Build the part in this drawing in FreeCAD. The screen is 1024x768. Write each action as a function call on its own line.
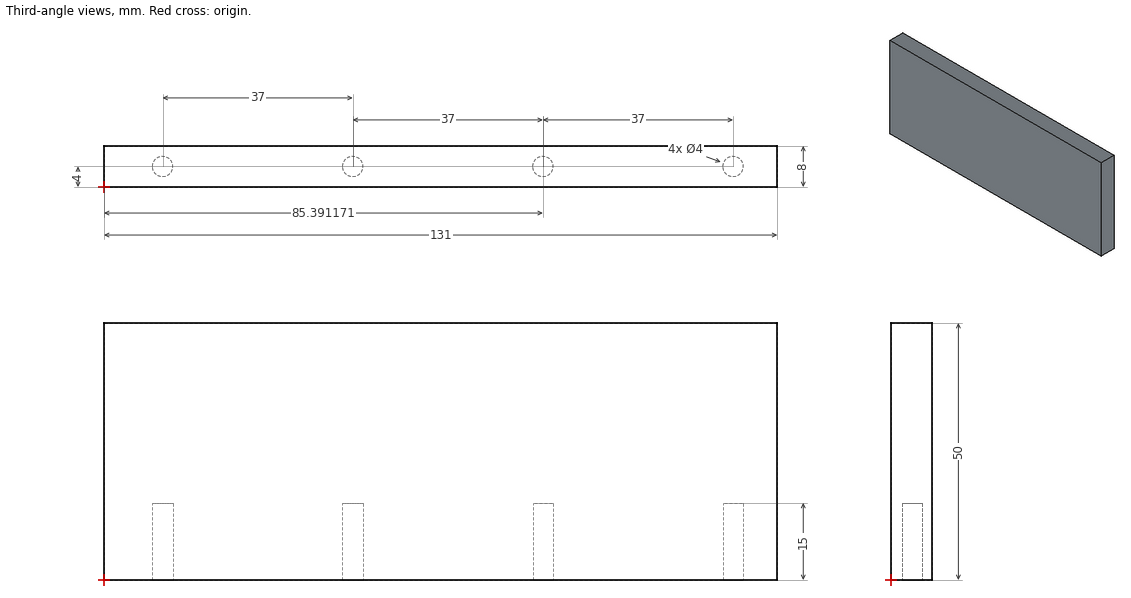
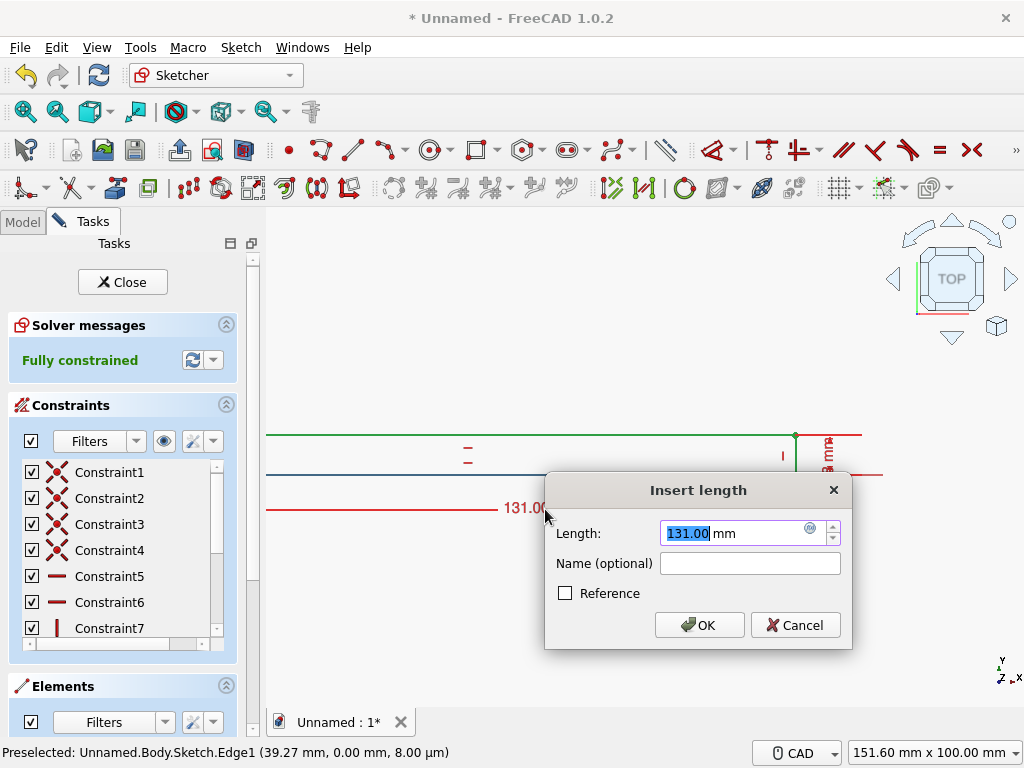
text(131)
key(Return)
key(Escape)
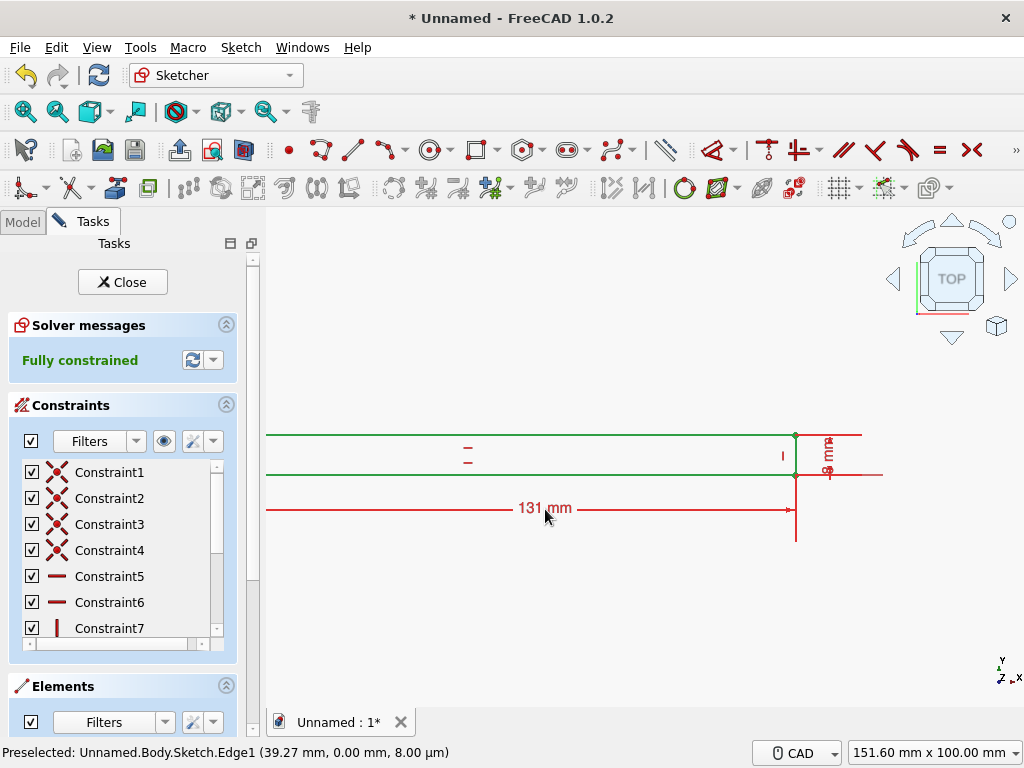
click(123, 282)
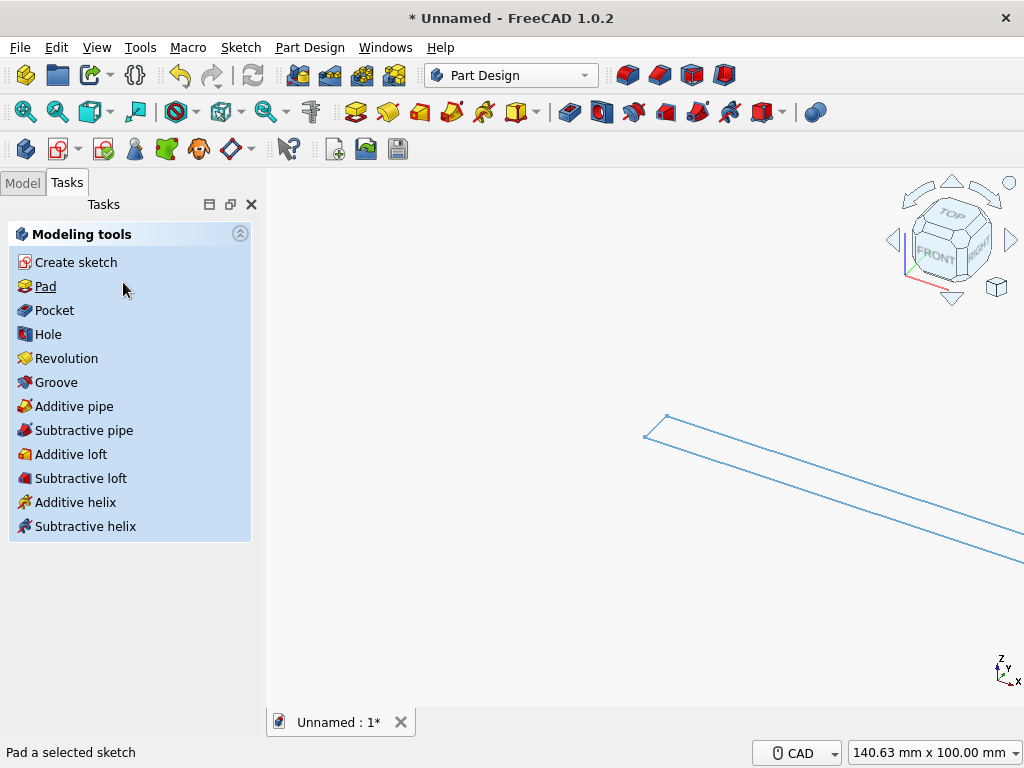
click(356, 112)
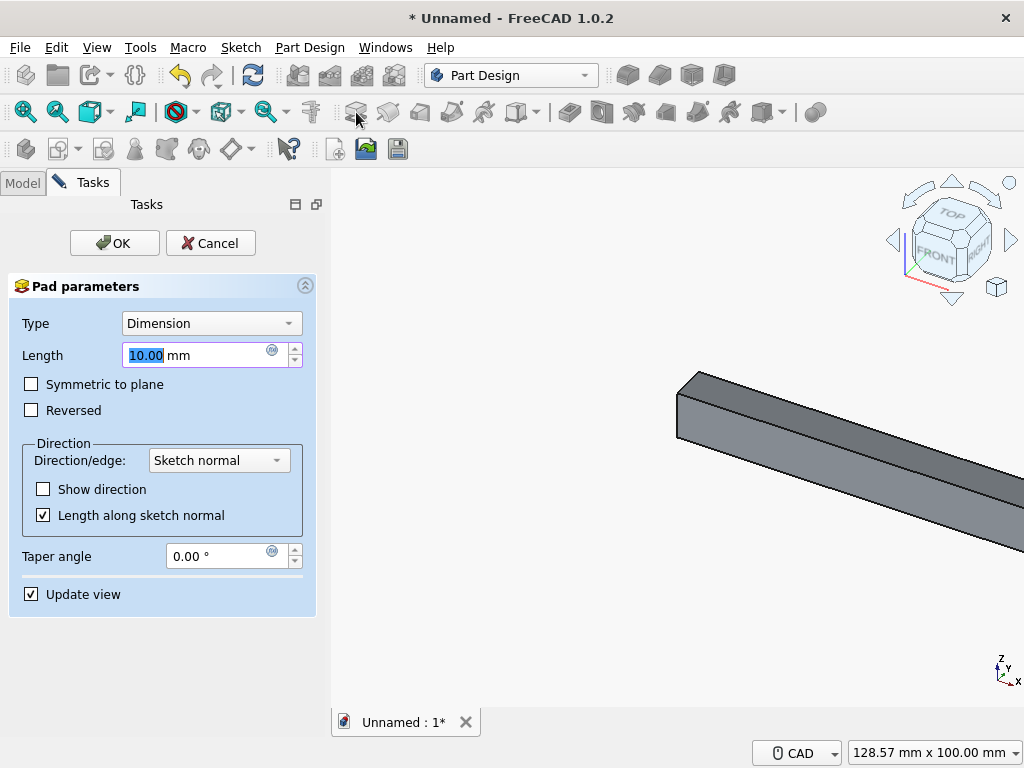
text(50)
key(Tab)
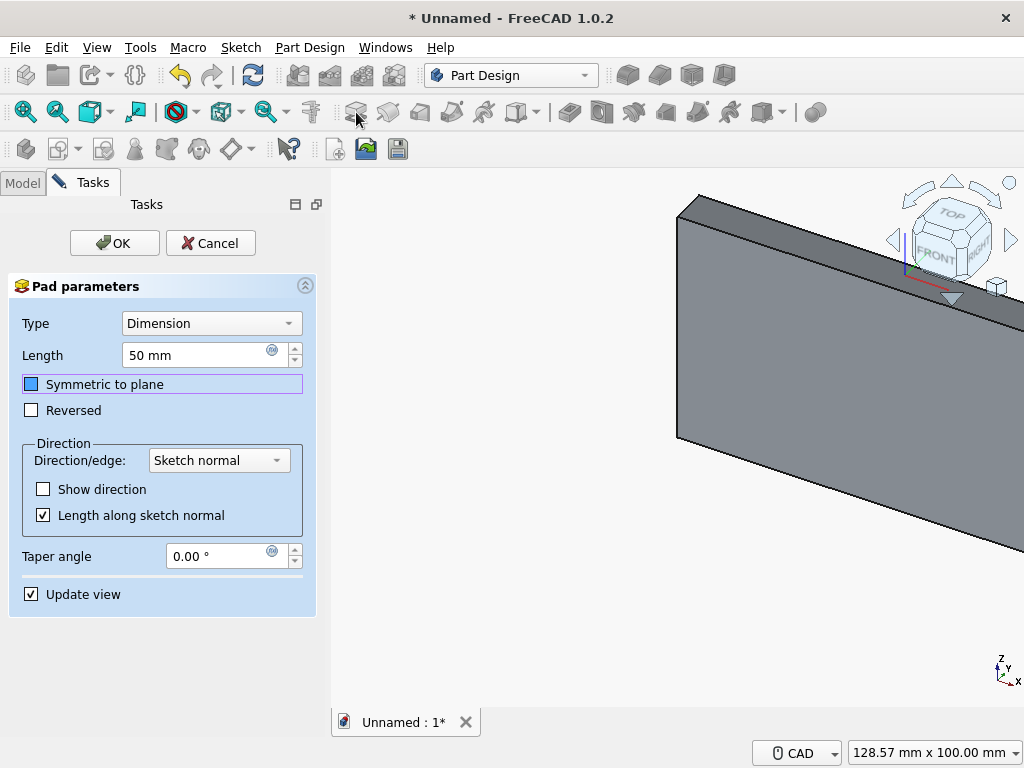
click(115, 243)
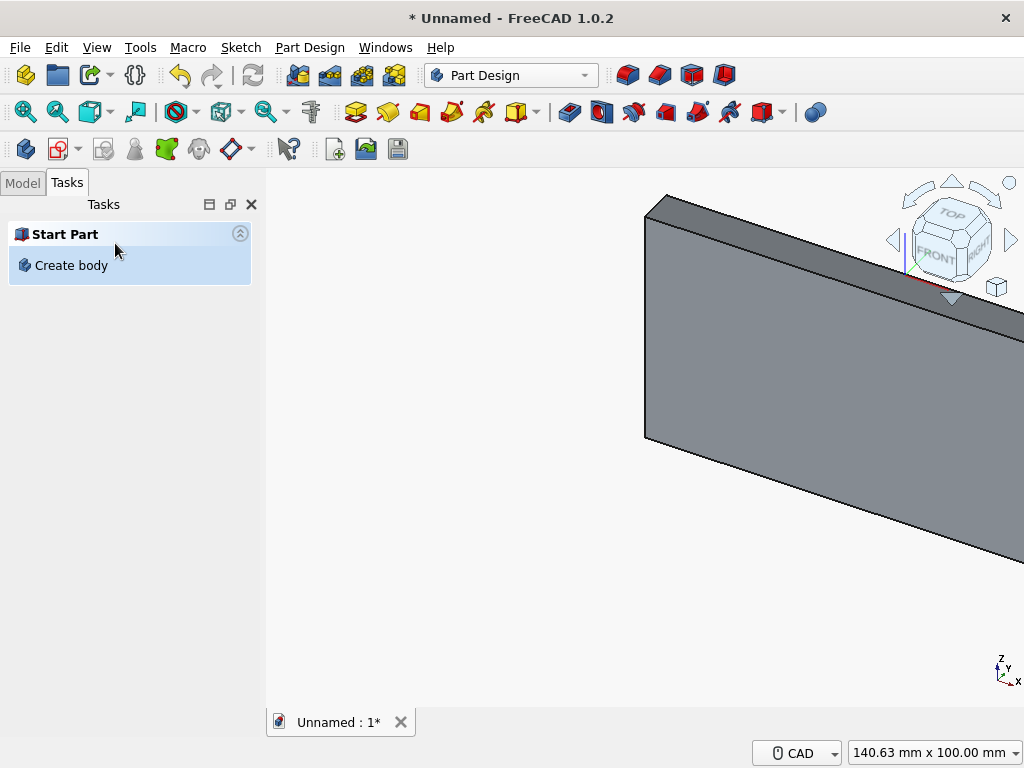
click(26, 112)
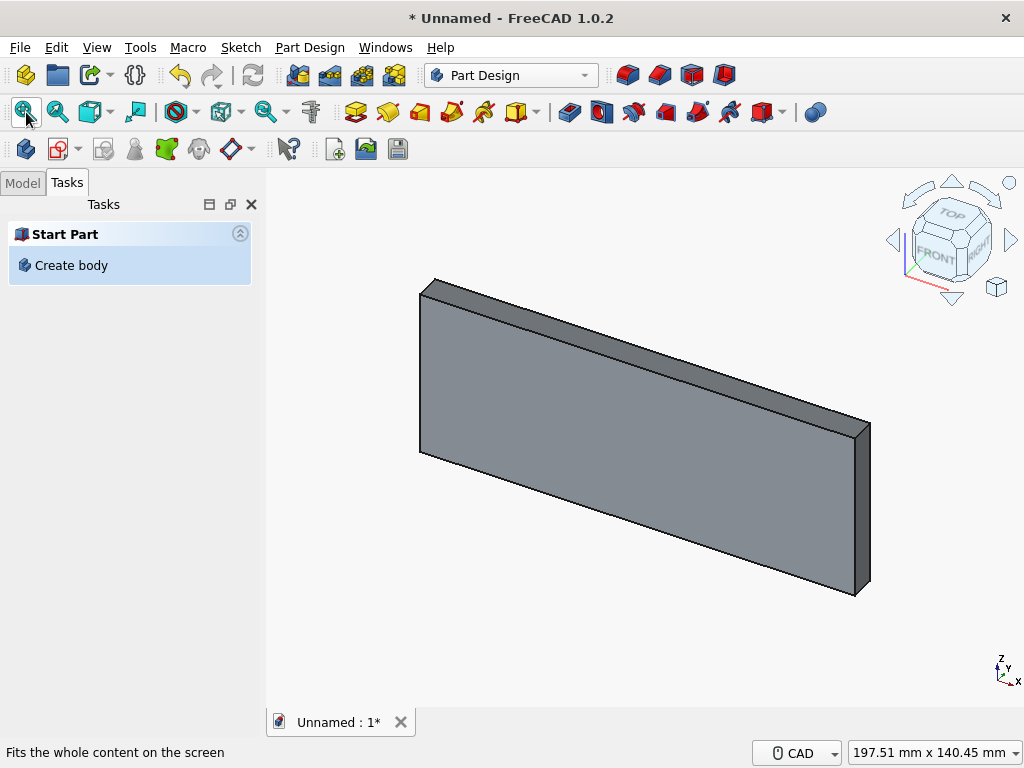
click(58, 150)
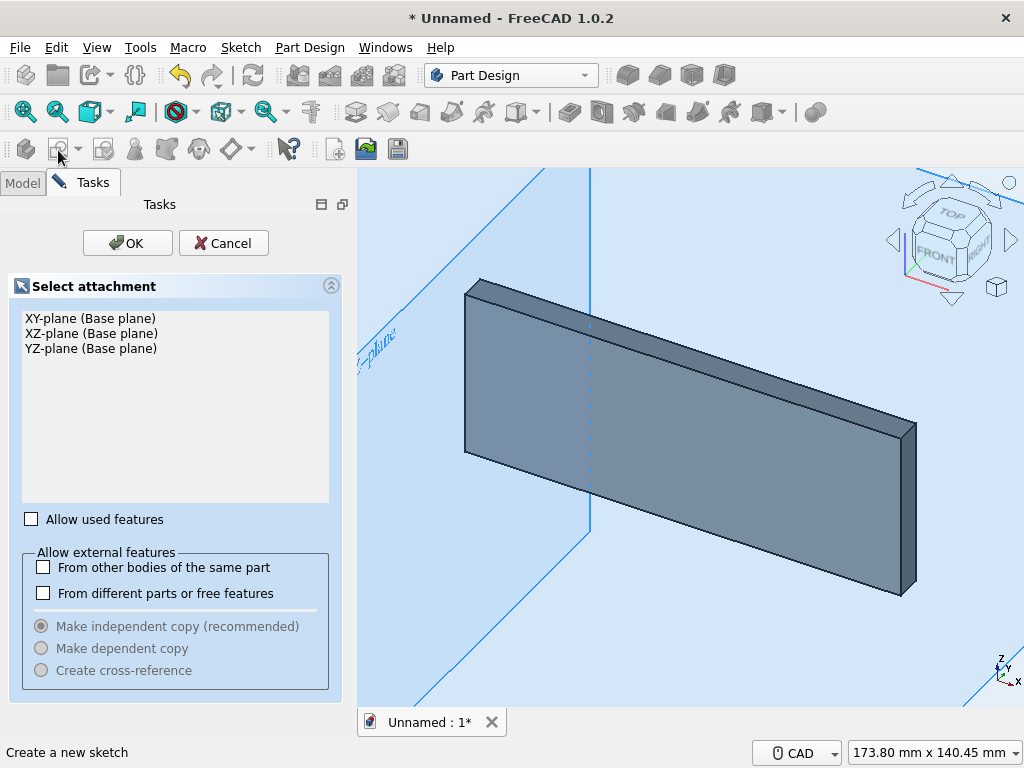
click(82, 318)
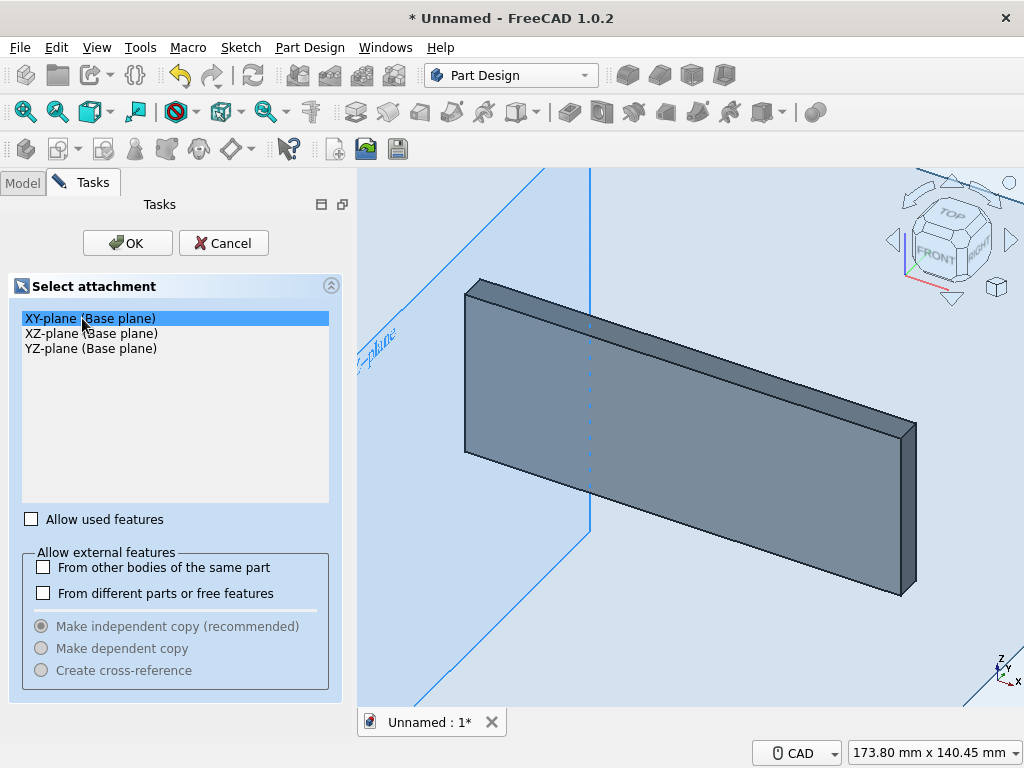
click(128, 243)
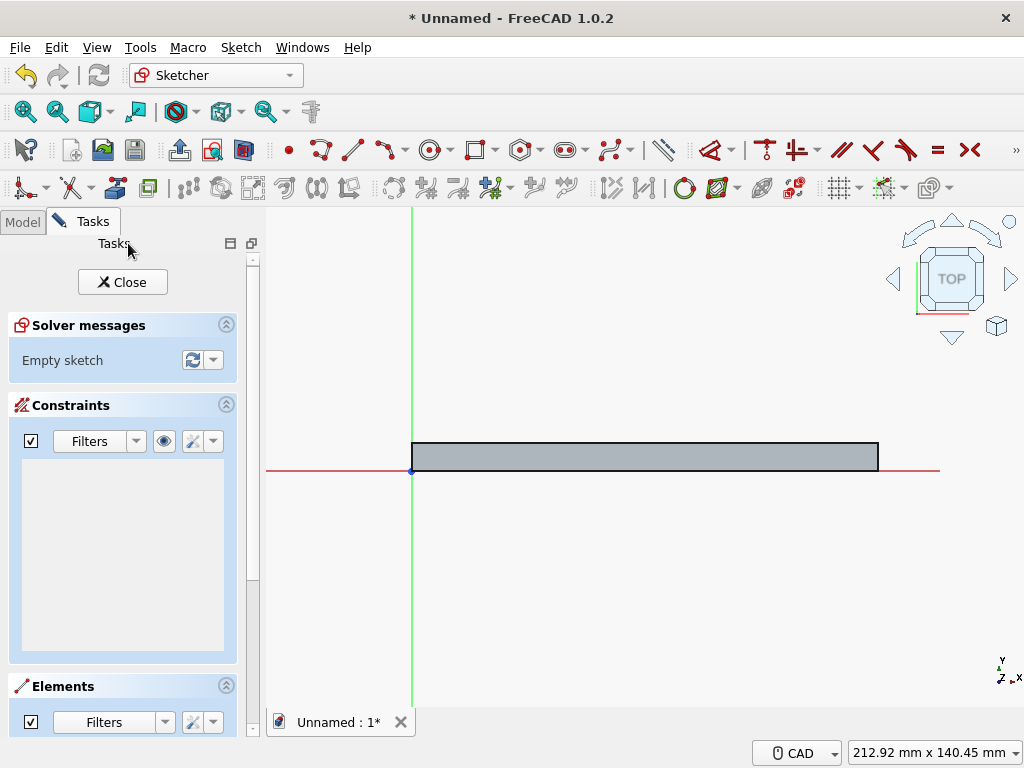
click(244, 150)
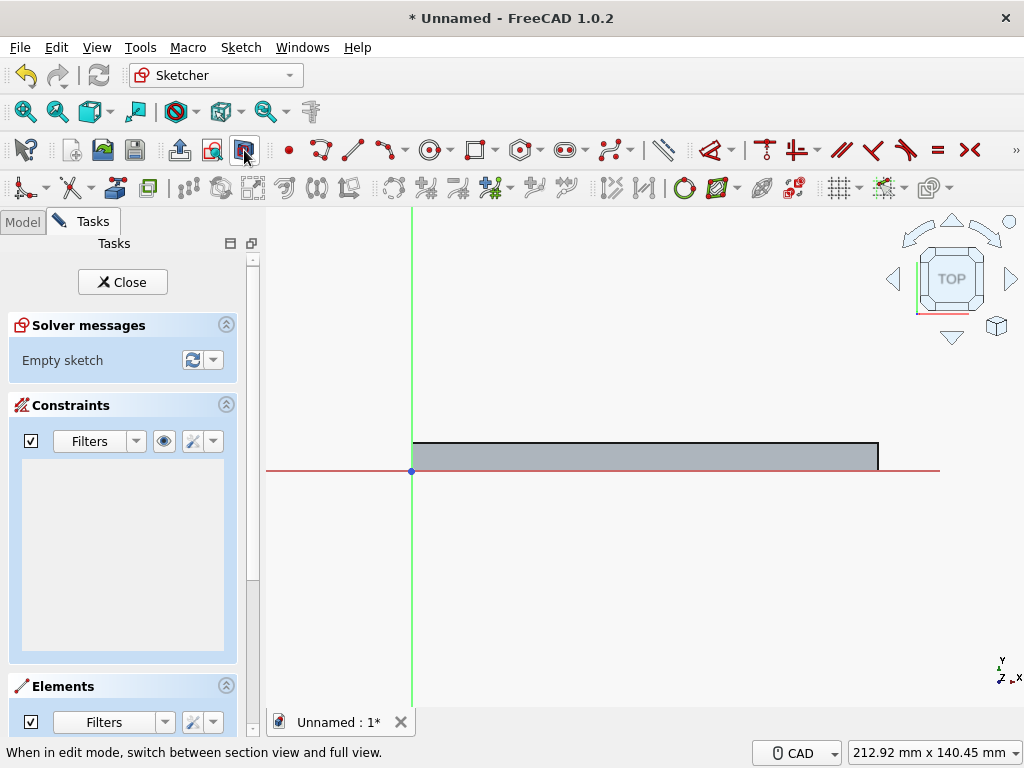
scroll(320, 441, down, 1)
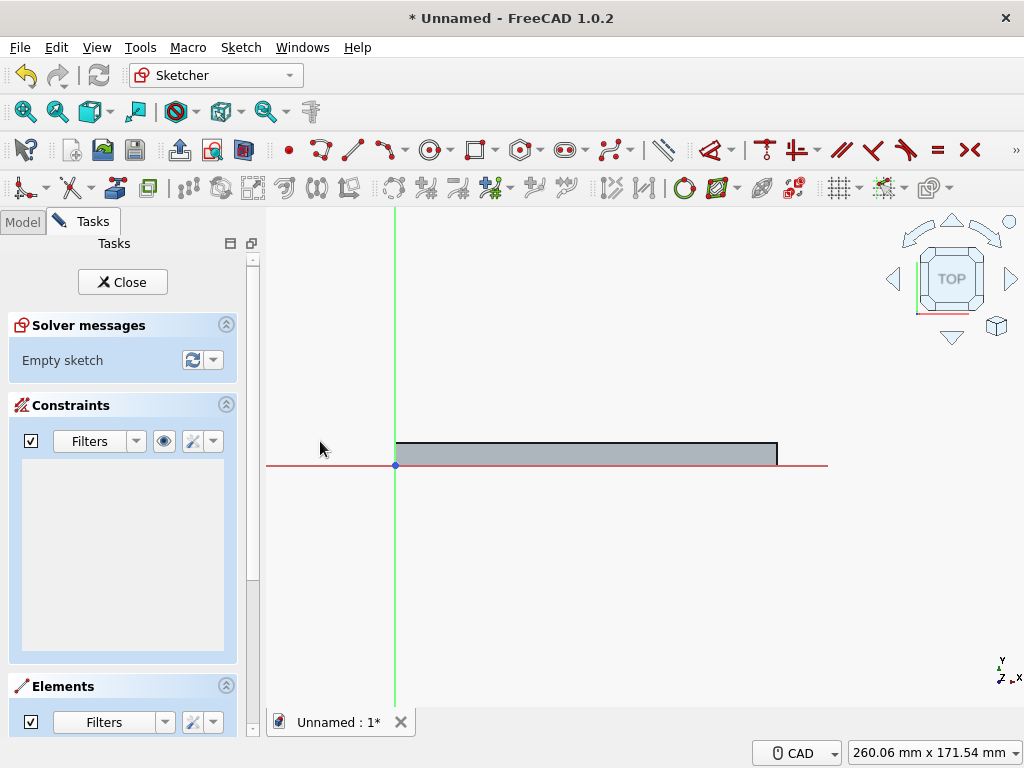
click(430, 150)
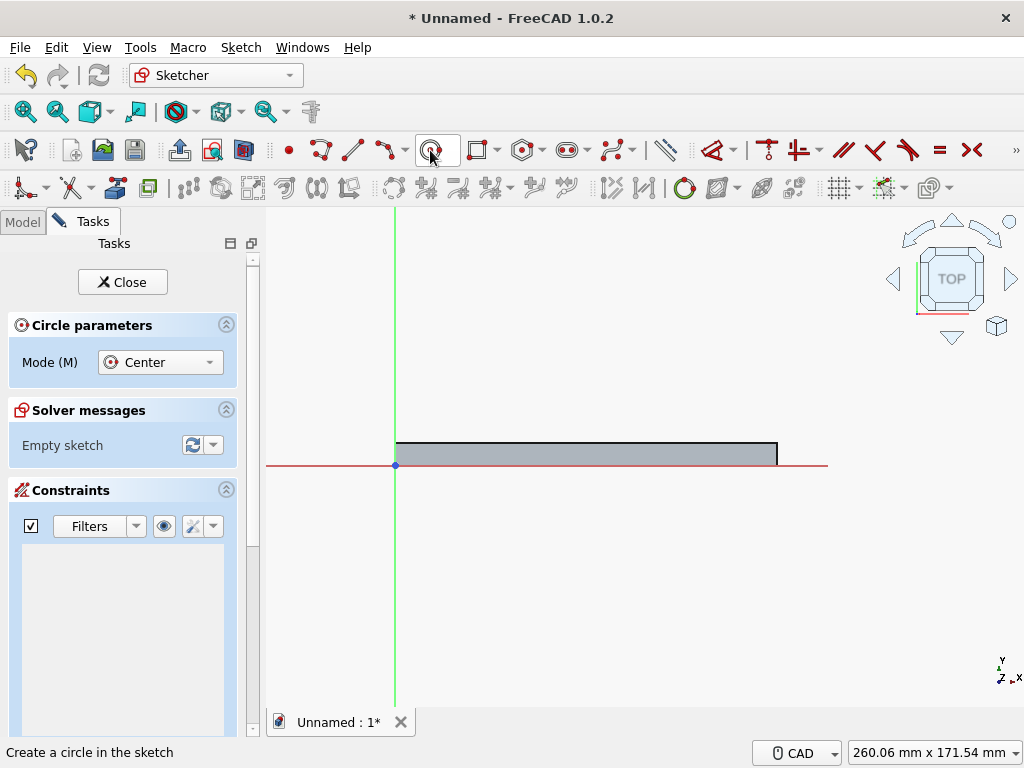
scroll(752, 454, up, 7)